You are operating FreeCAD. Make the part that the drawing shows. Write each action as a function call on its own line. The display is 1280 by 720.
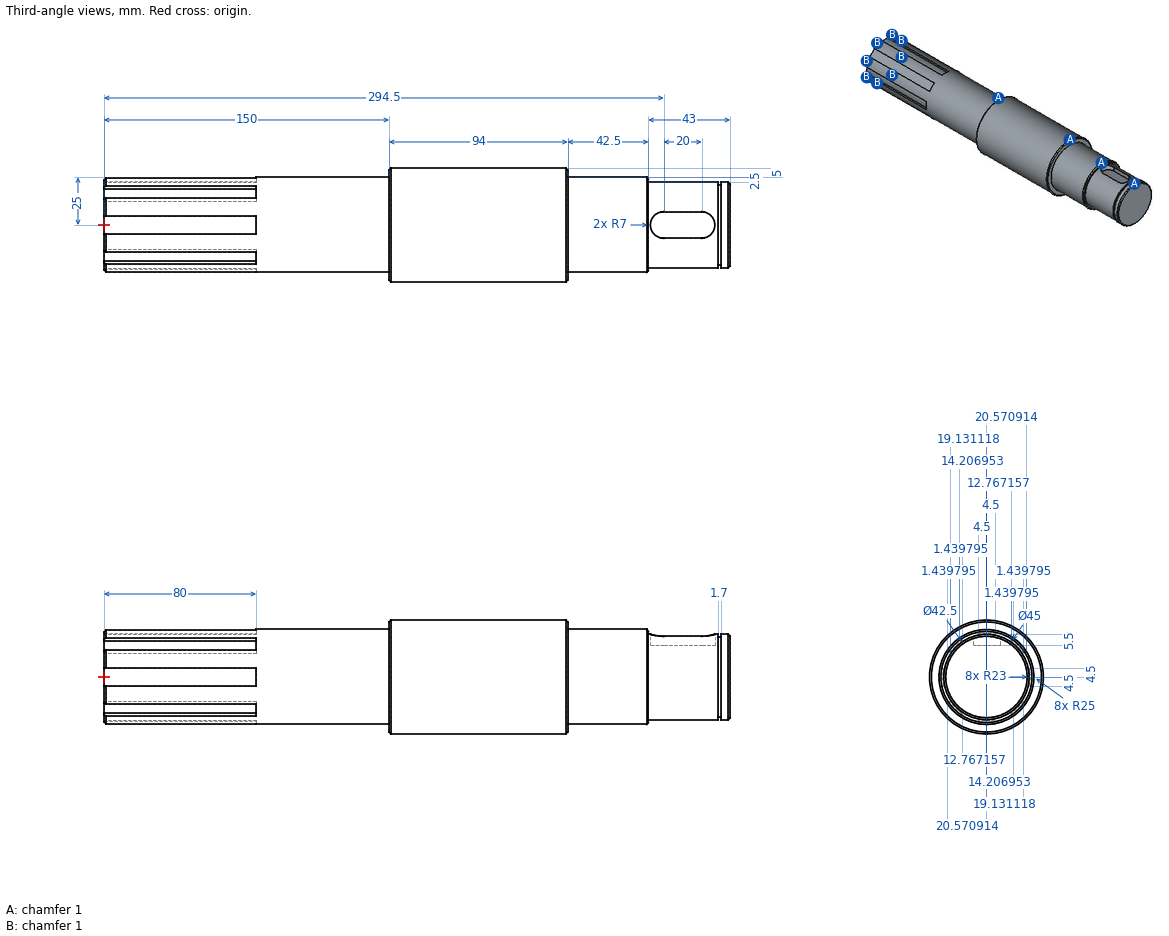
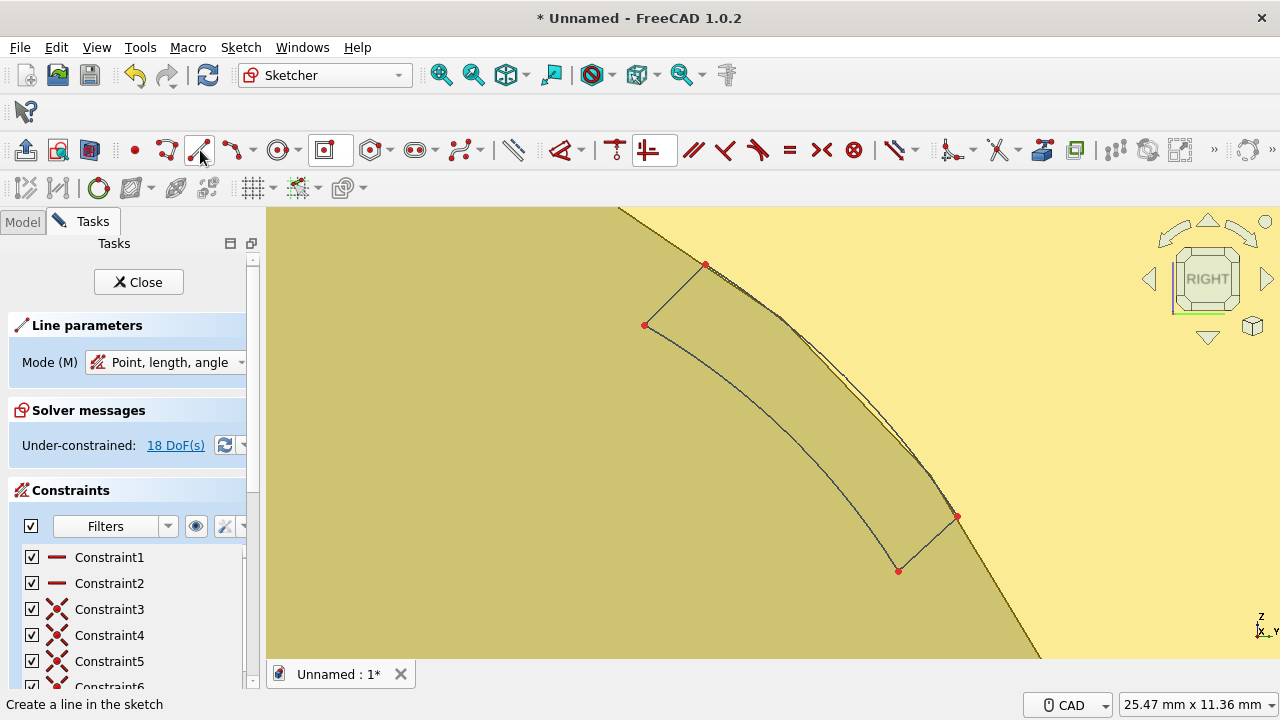
scroll(793, 332, down, 10)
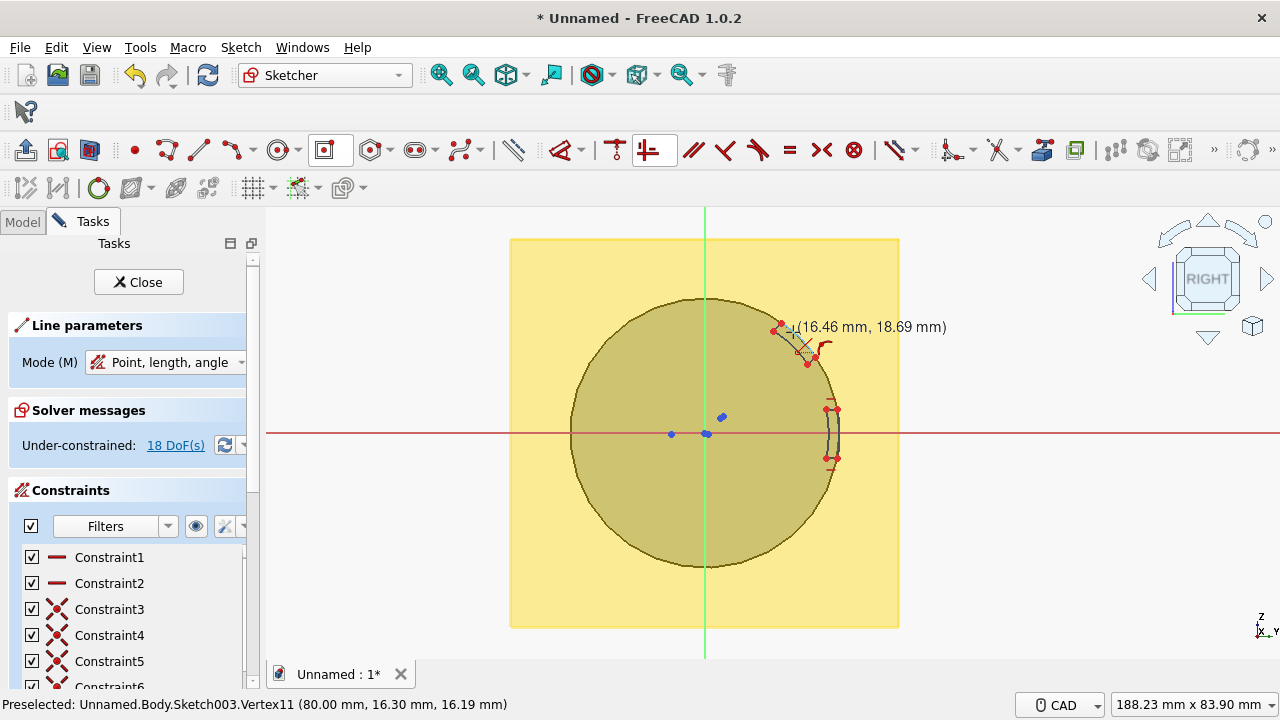
click(681, 312)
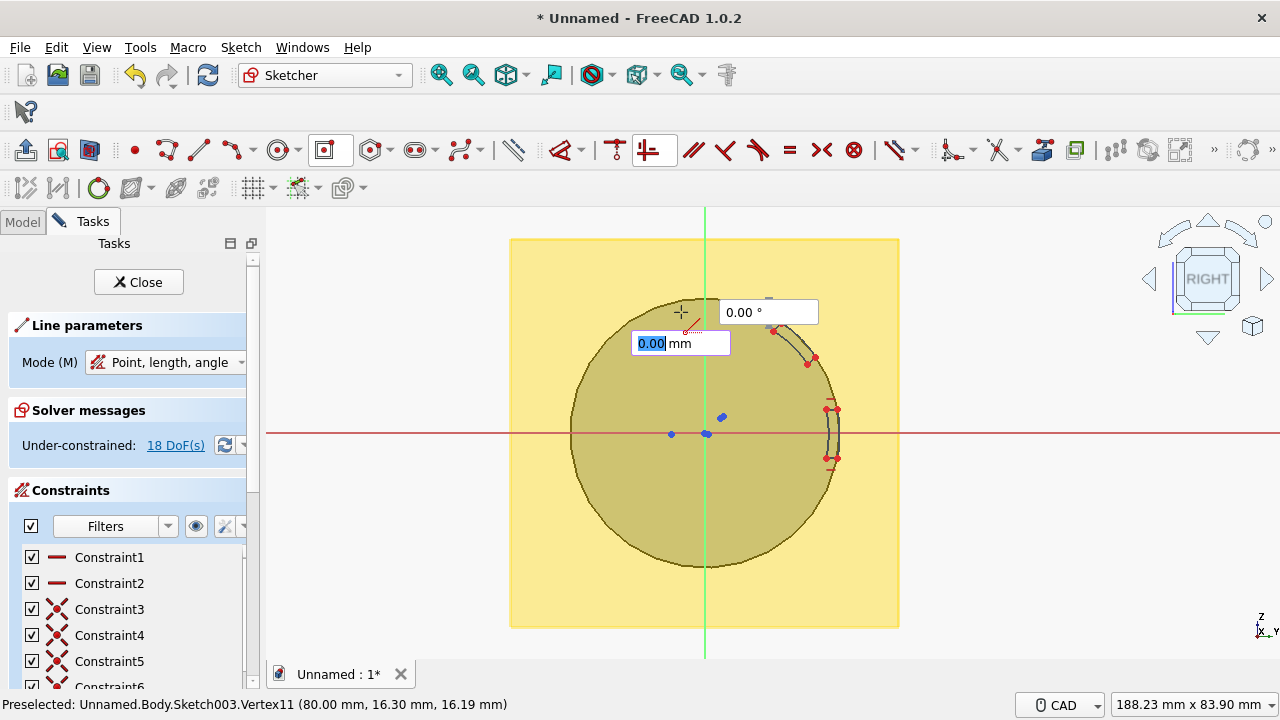
scroll(681, 301, up, 2)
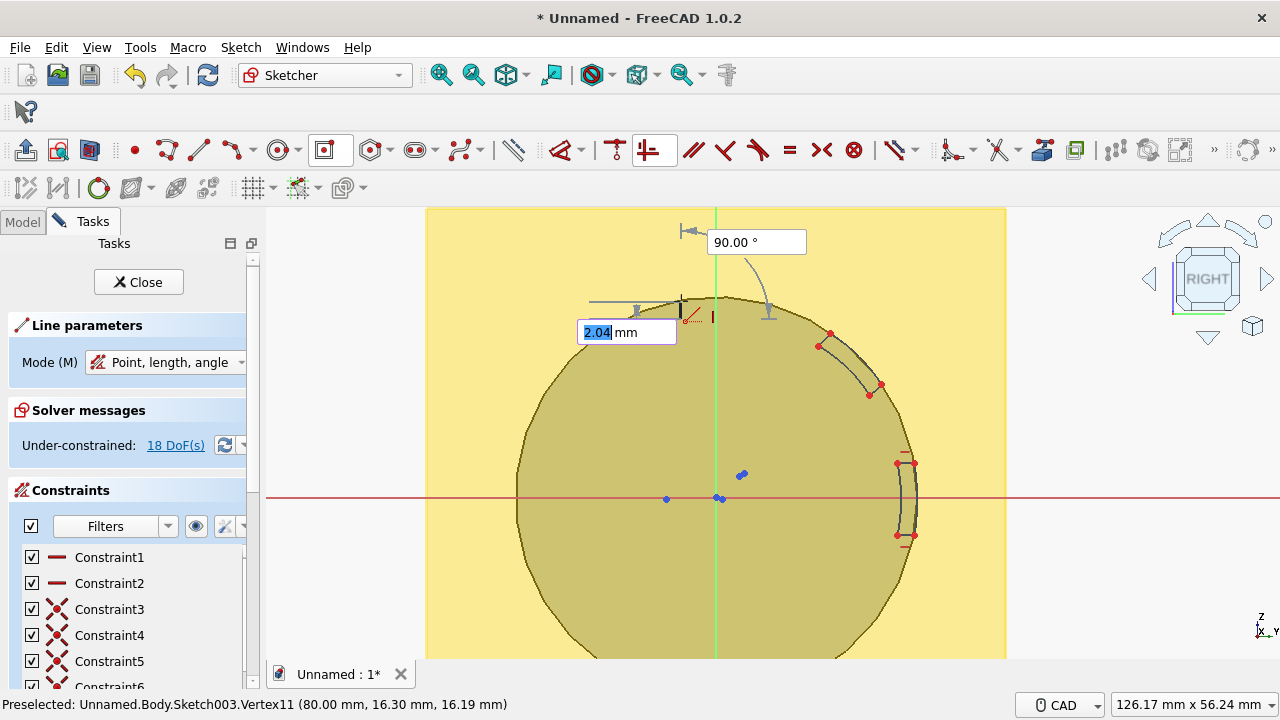
click(681, 300)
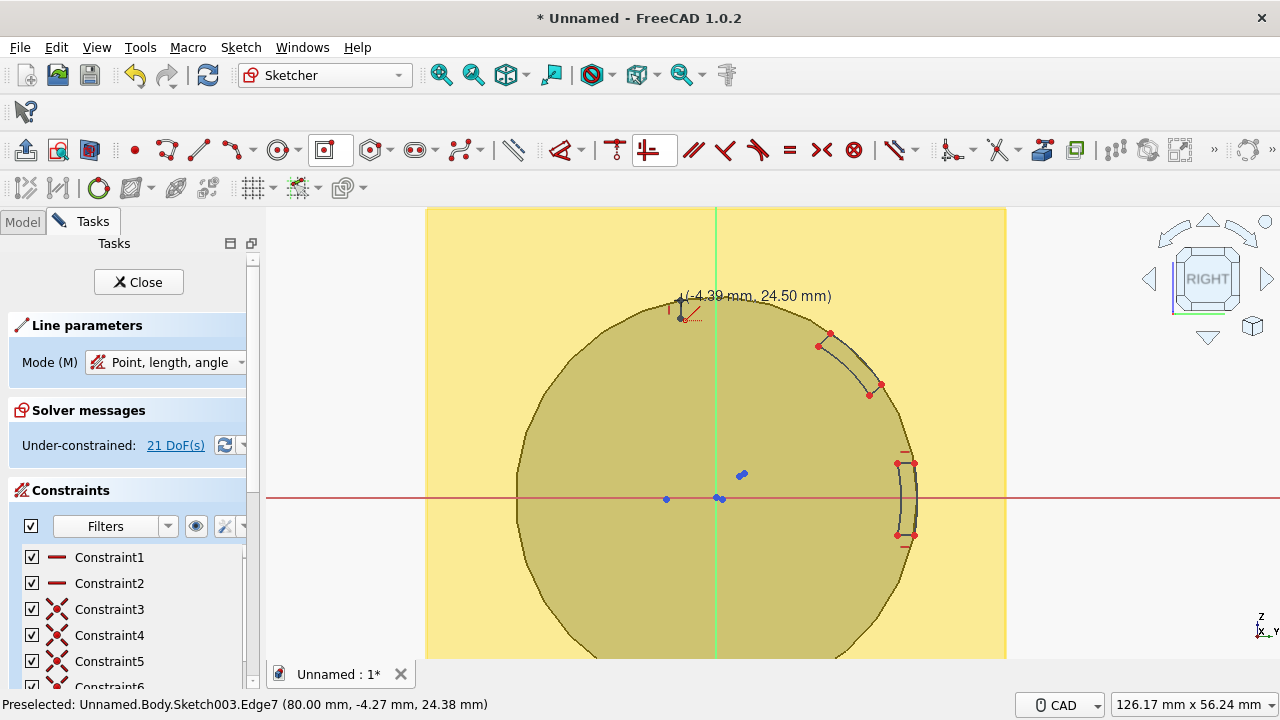
click(752, 300)
click(752, 317)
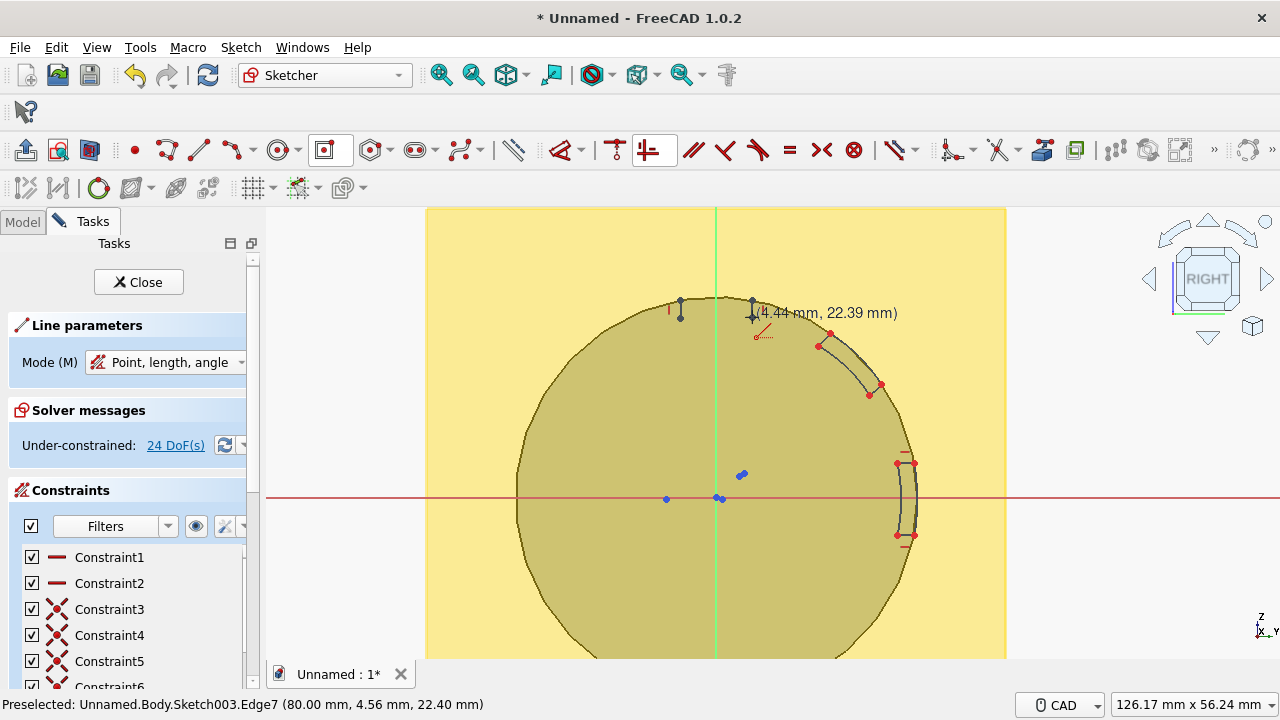
click(232, 150)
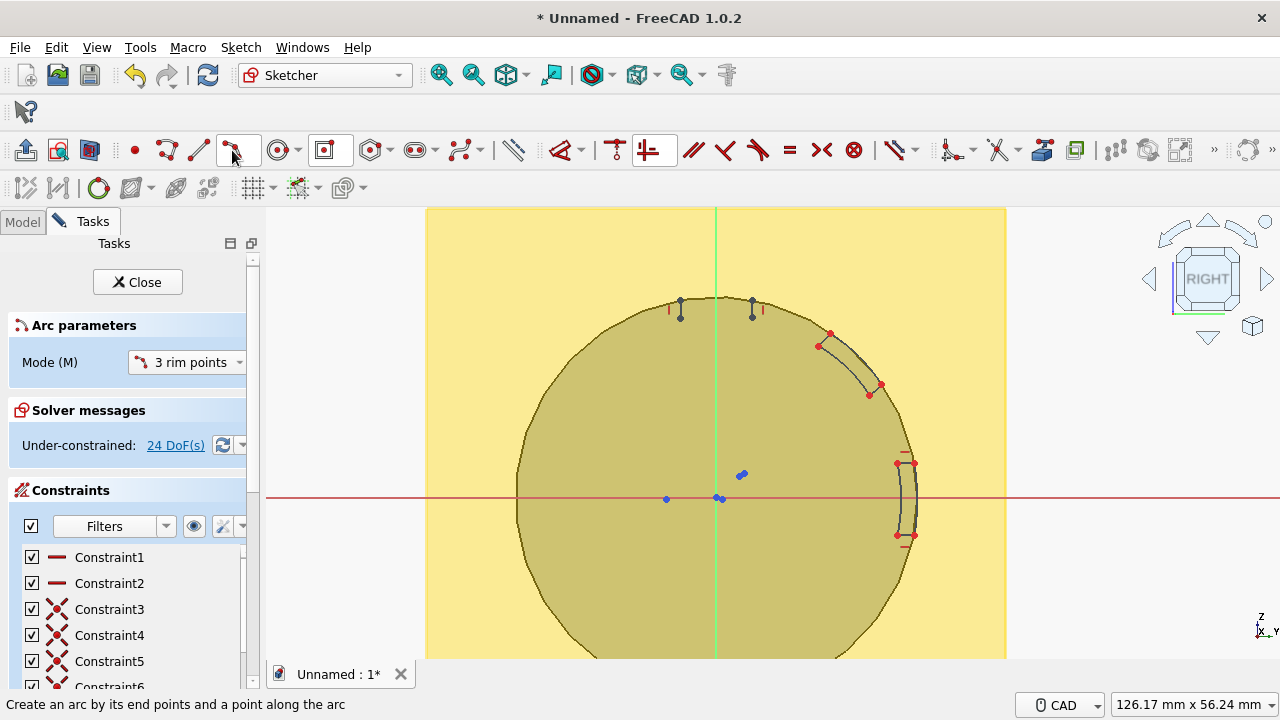
scroll(680, 300, up, 4)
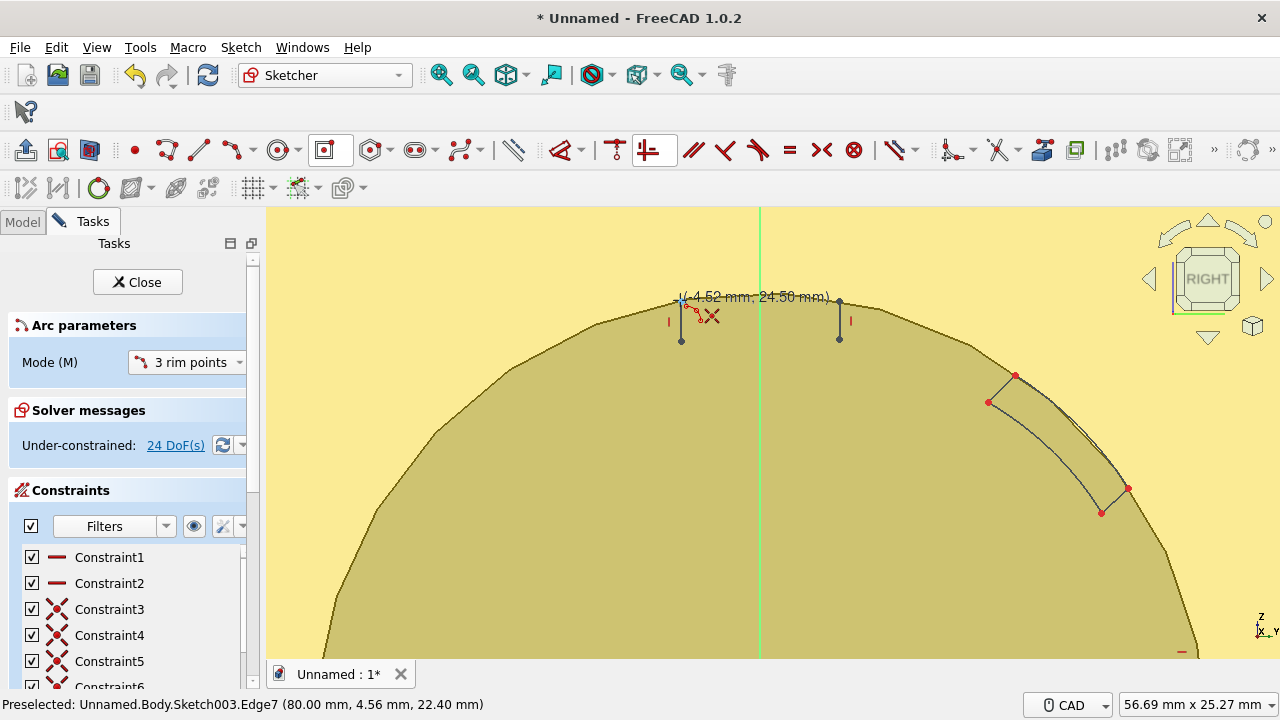
click(681, 302)
click(840, 302)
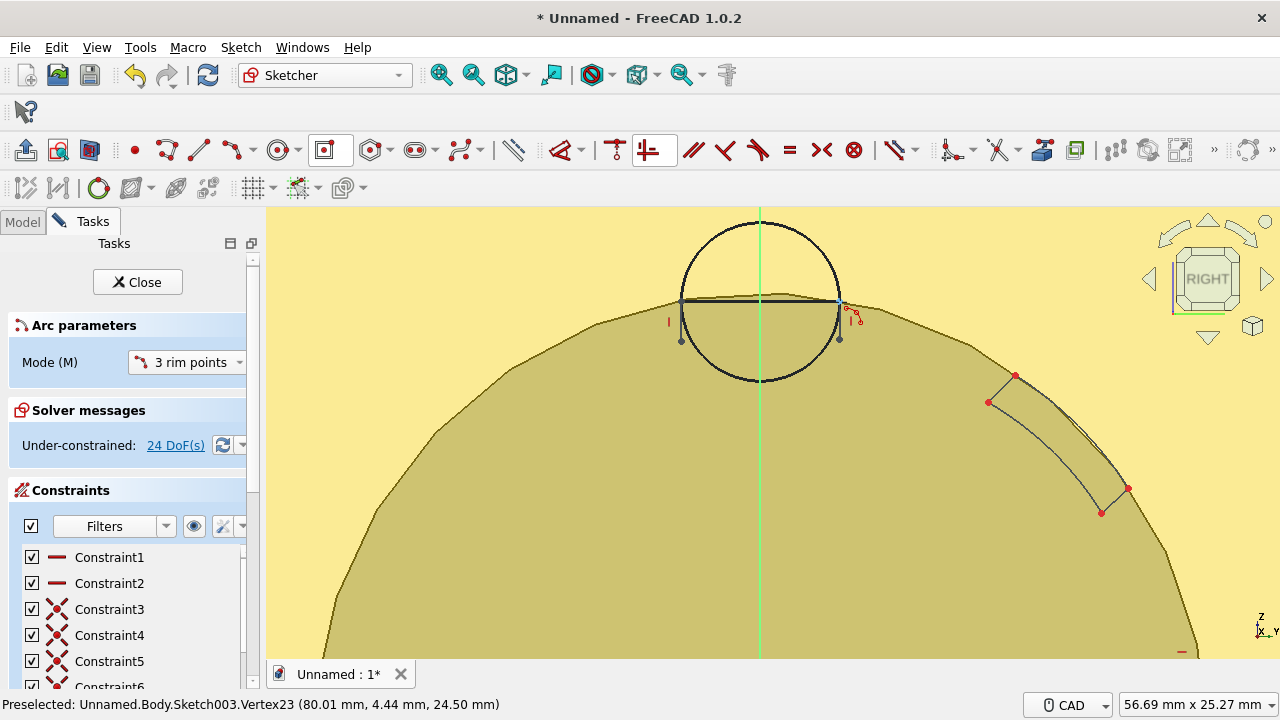
scroll(776, 293, up, 5)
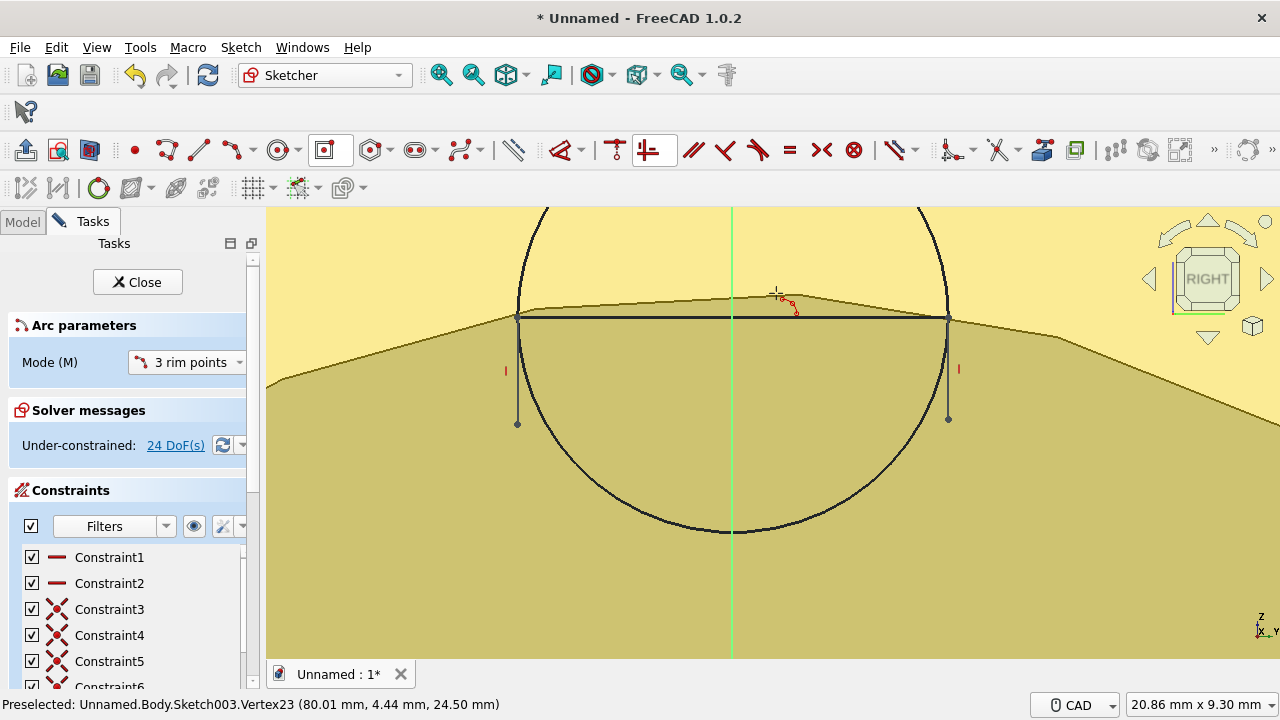
click(776, 294)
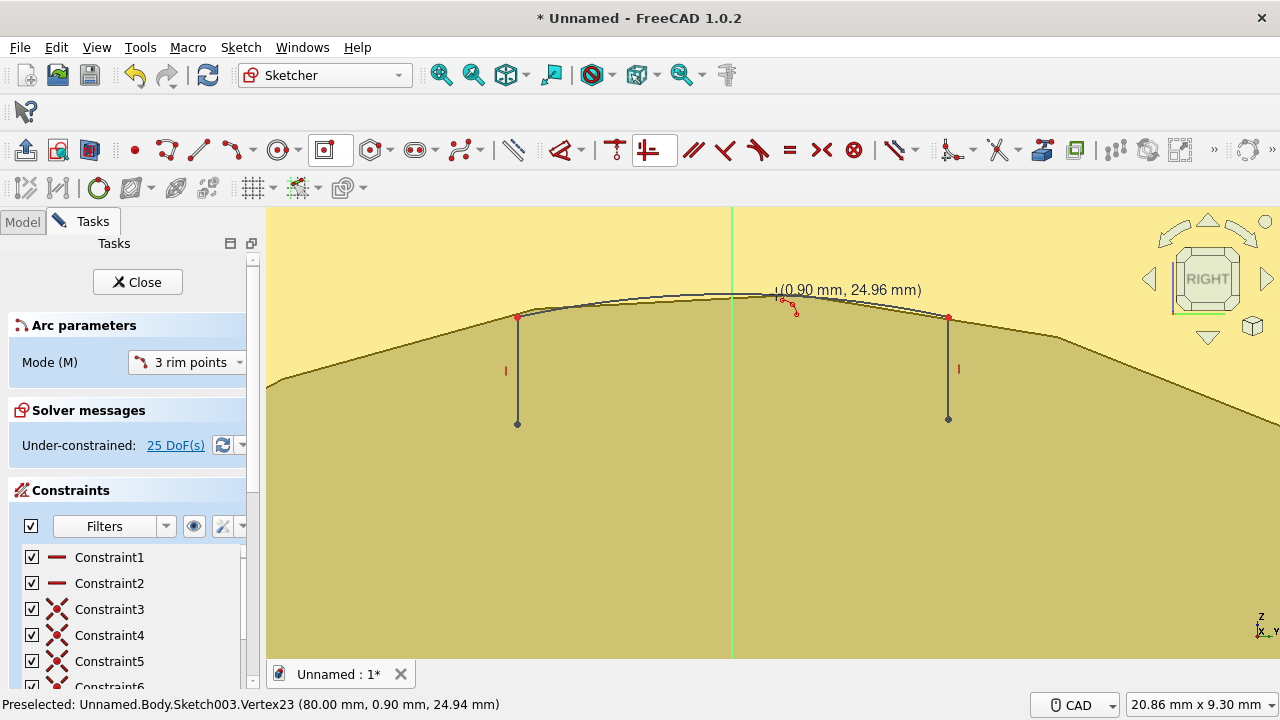
scroll(701, 299, down, 11)